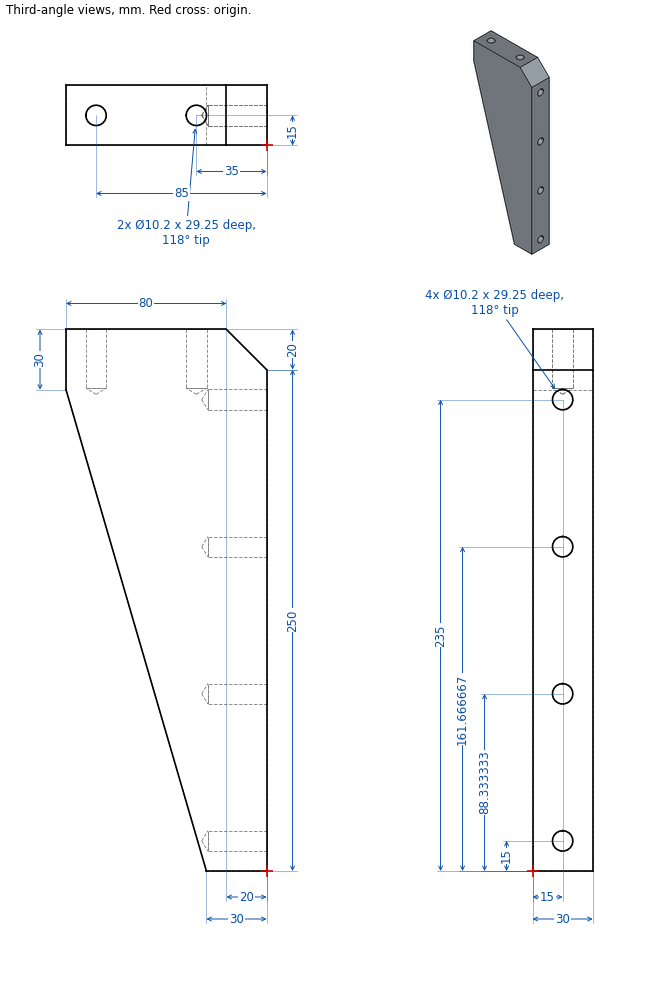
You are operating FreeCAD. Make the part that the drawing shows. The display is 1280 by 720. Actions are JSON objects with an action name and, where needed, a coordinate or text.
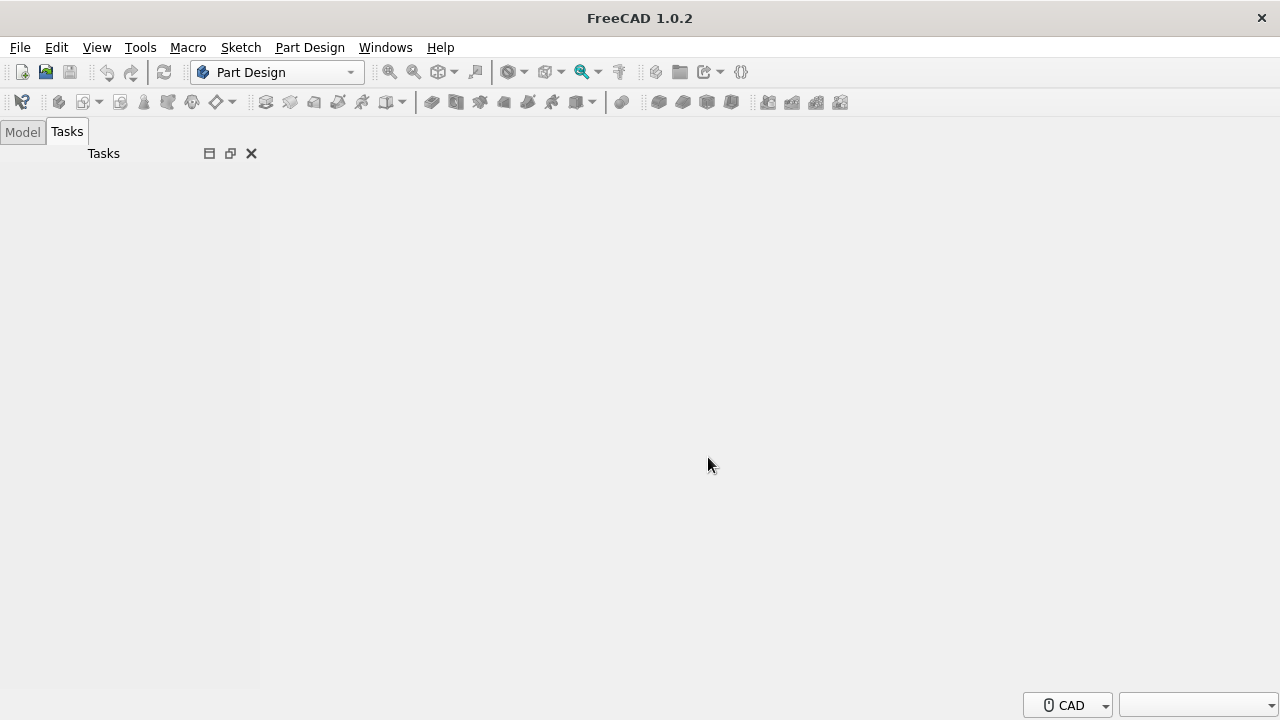
{"action": "key", "text": "ctrl+n"}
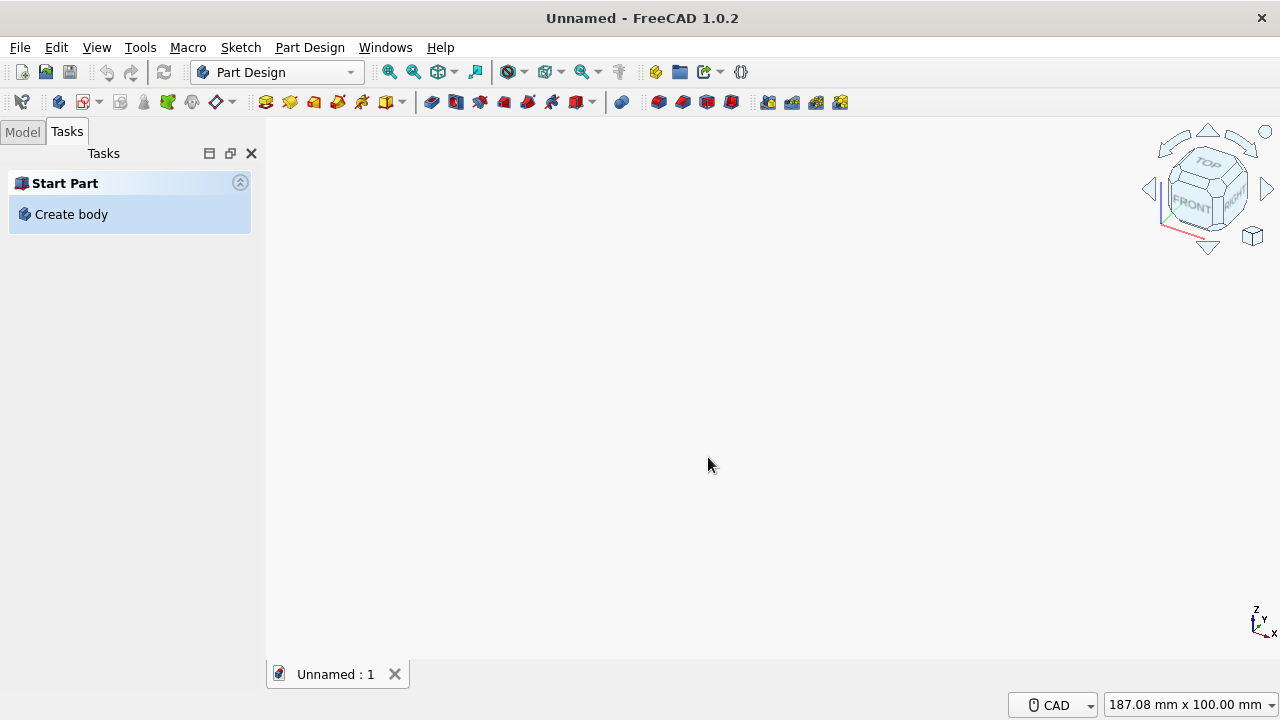
{"action": "left_click", "coordinate": [84, 102]}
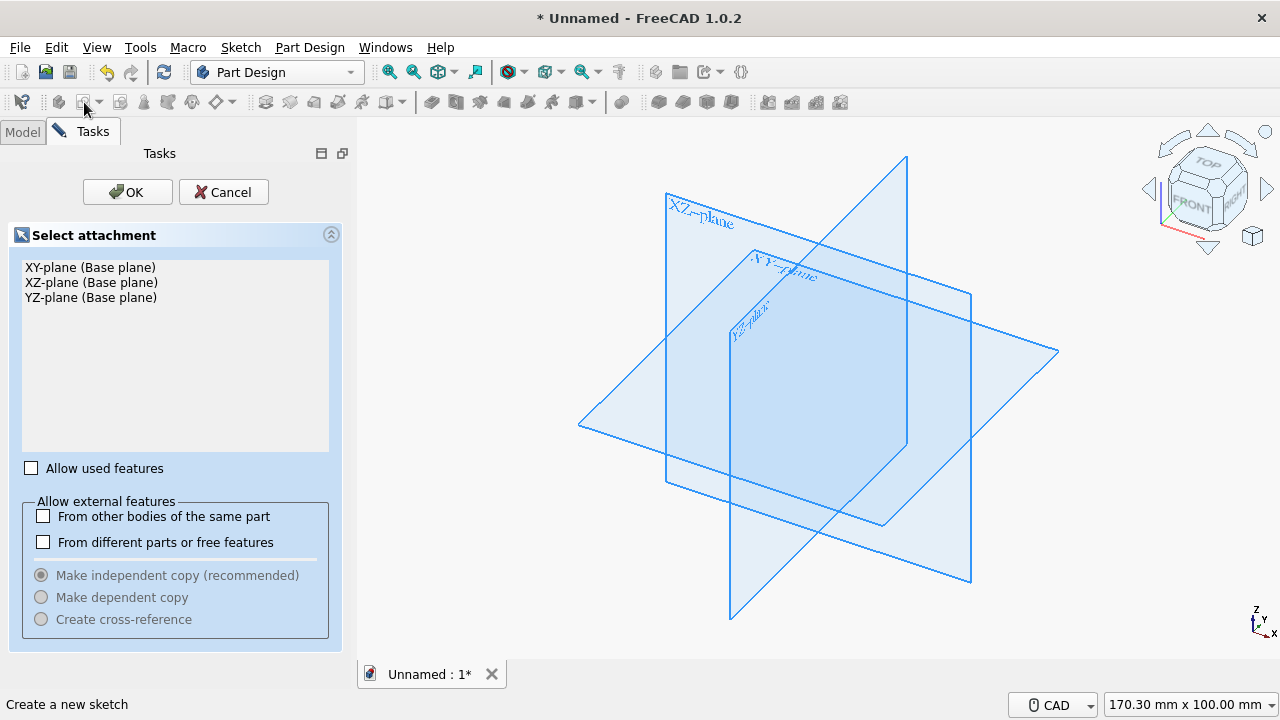
{"action": "left_click", "coordinate": [82, 282]}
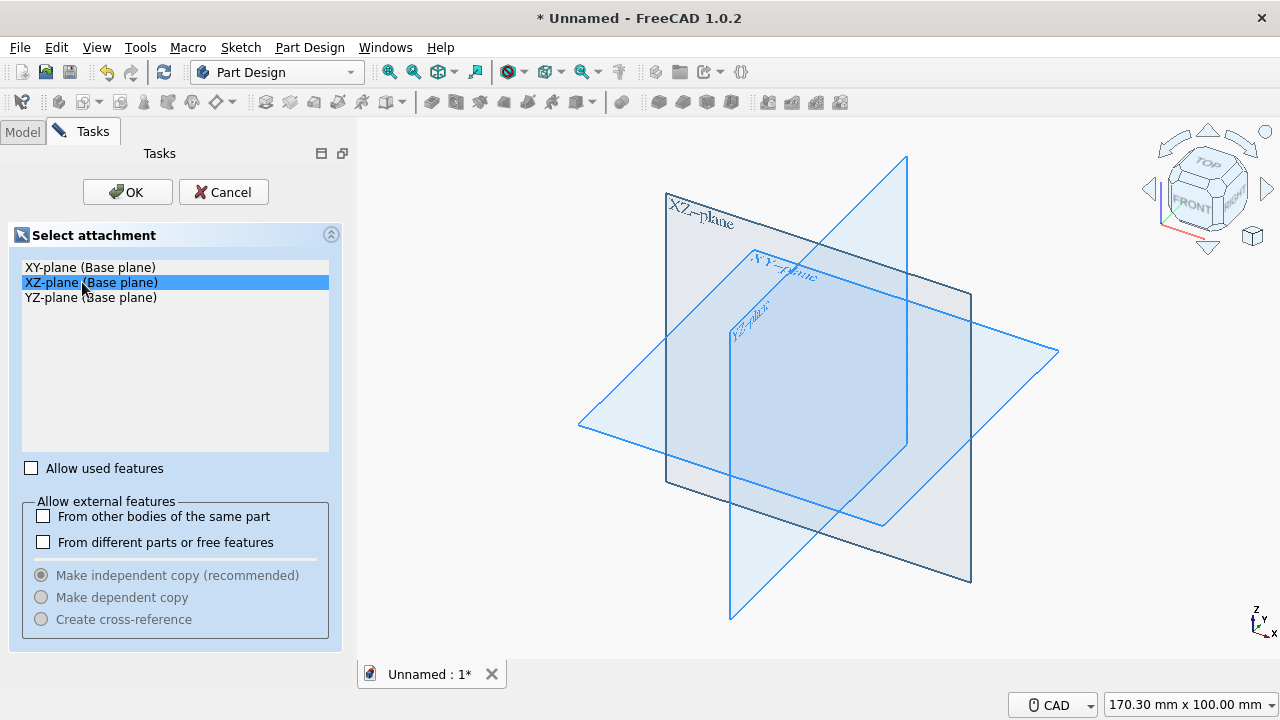
{"action": "left_click", "coordinate": [128, 192]}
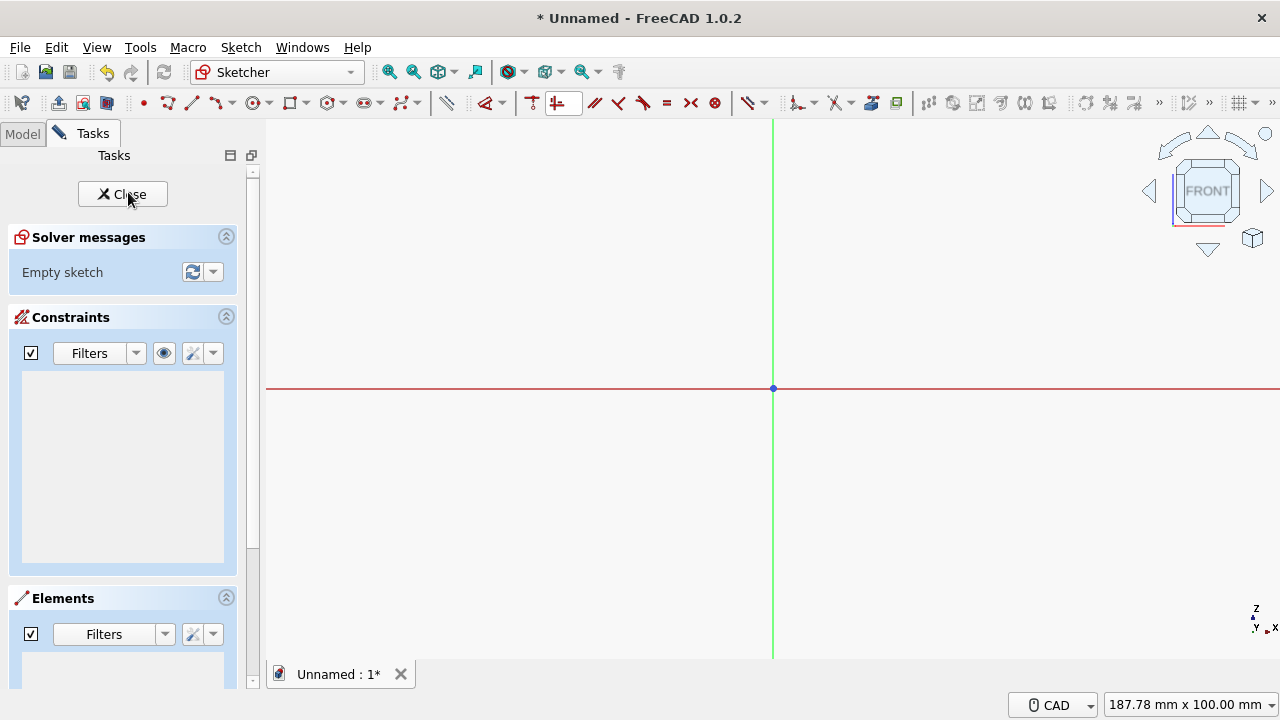
{"action": "scroll", "coordinate": [770, 628], "scroll_direction": "down", "scroll_amount": 7}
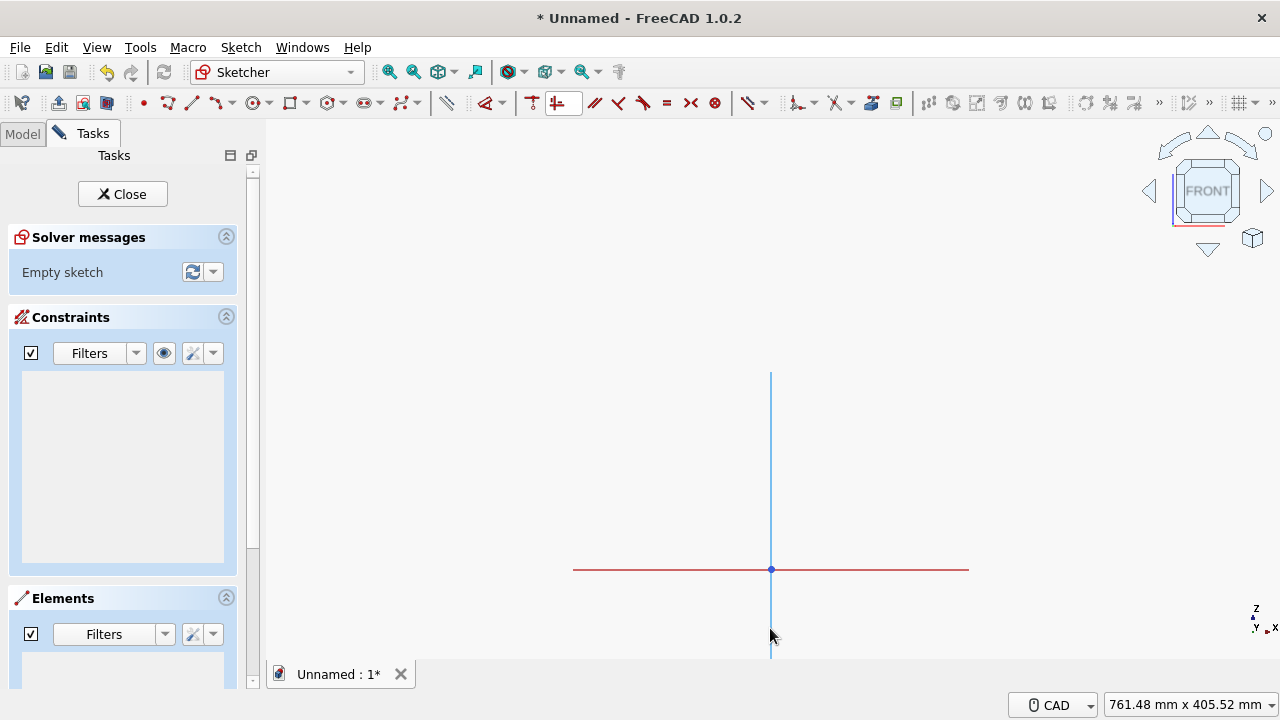
{"action": "key", "text": "g m"}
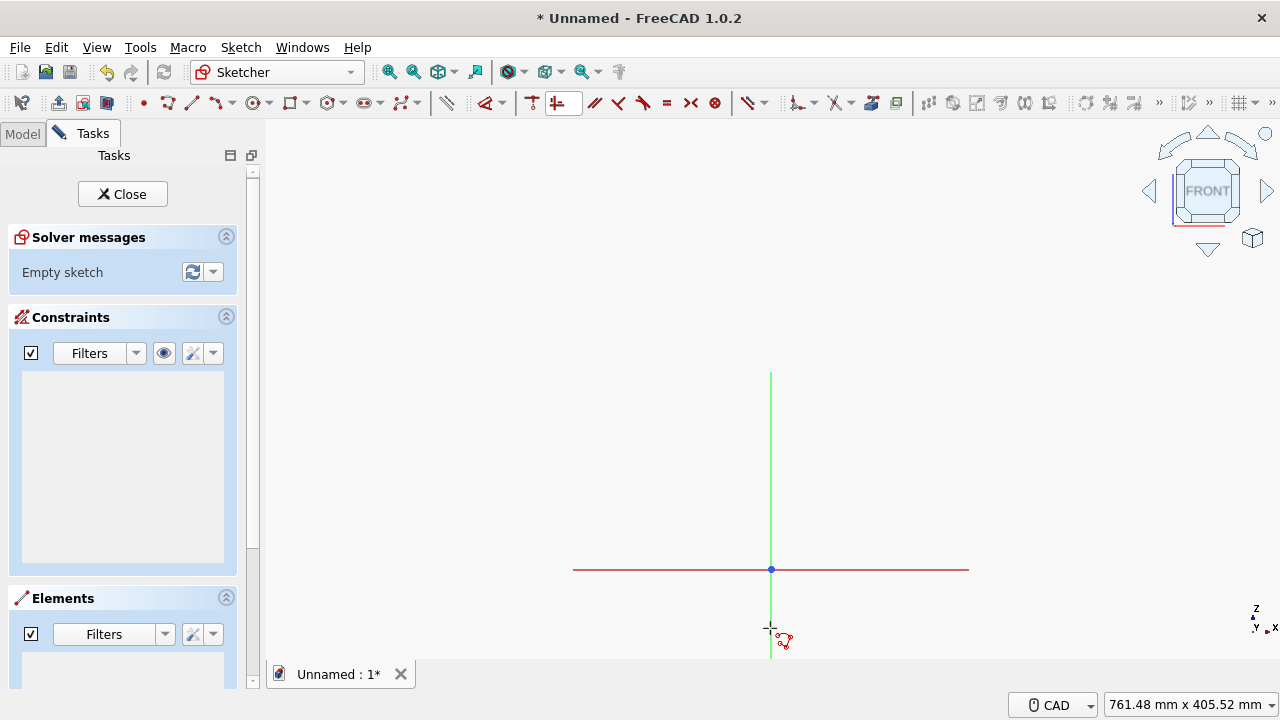
{"action": "left_click", "coordinate": [771, 570]}
{"action": "left_click", "coordinate": [731, 561]}
{"action": "left_click", "coordinate": [638, 250]}
{"action": "left_click", "coordinate": [638, 210]}
{"action": "left_click", "coordinate": [744, 210]}
{"action": "left_click", "coordinate": [762, 237]}
{"action": "left_click", "coordinate": [771, 570]}
{"action": "key", "text": "Escape"}
{"action": "key", "text": "Escape"}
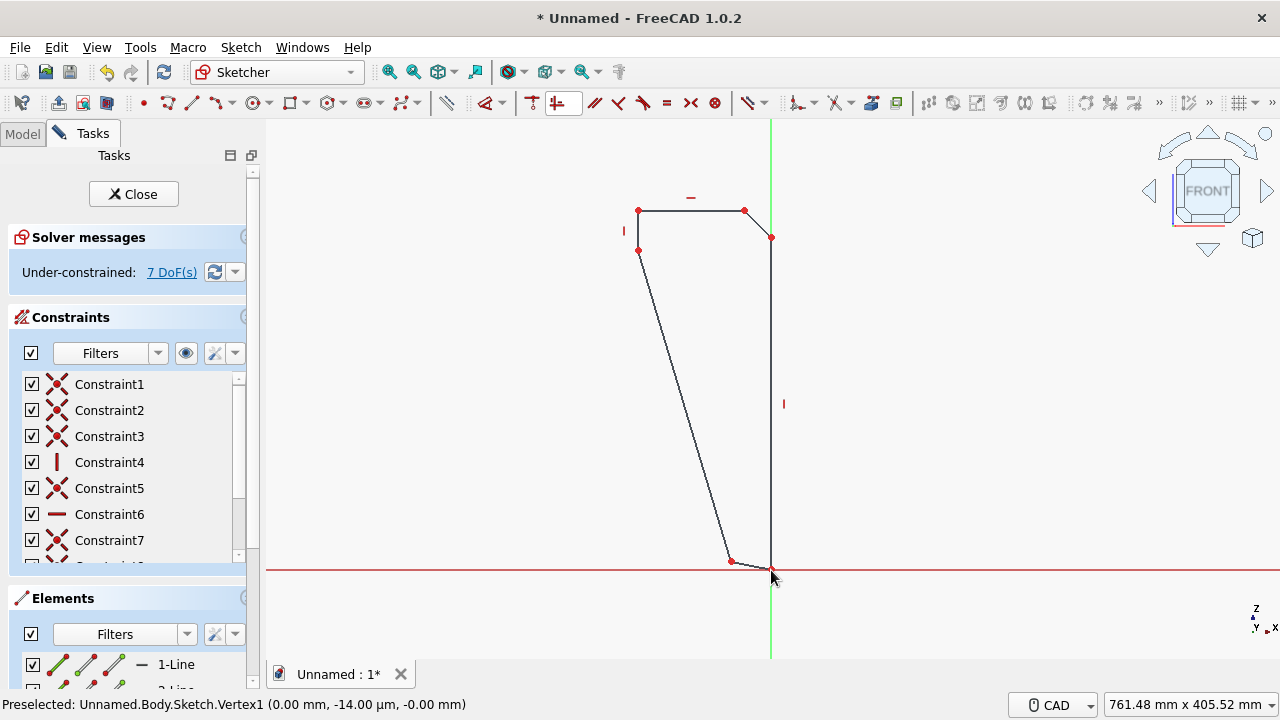
{"action": "left_click", "coordinate": [759, 567]}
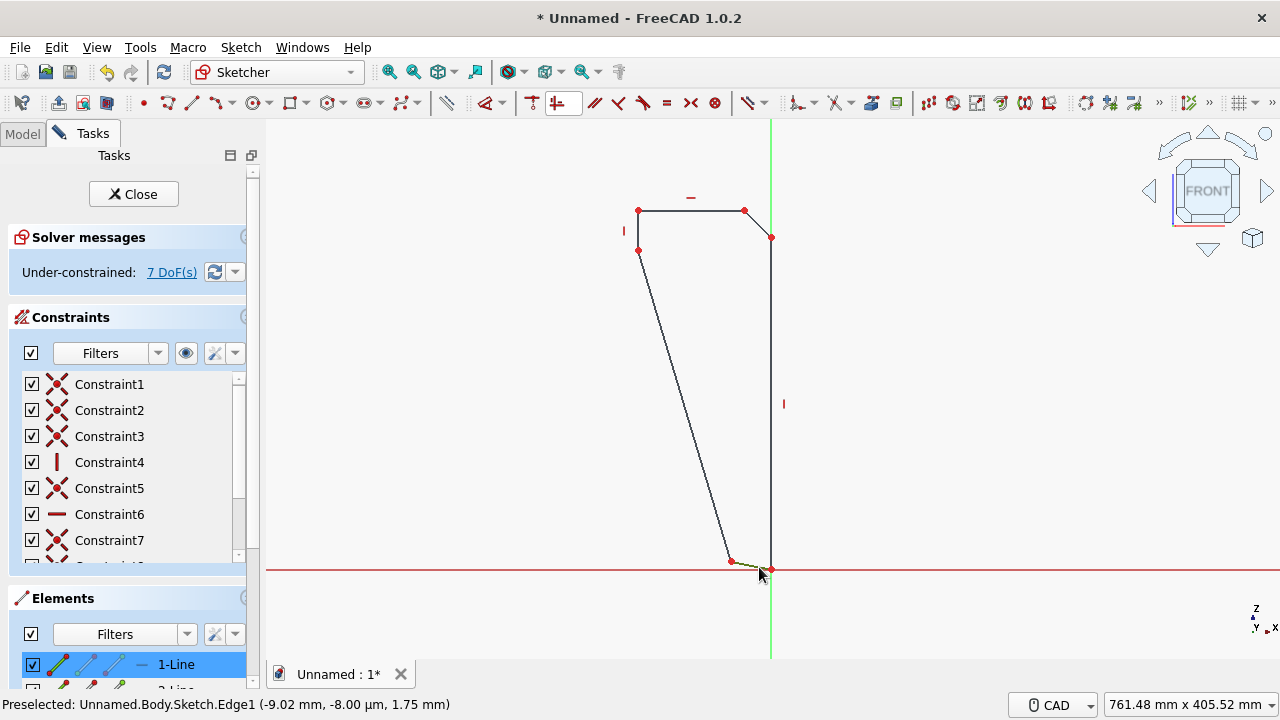
{"action": "key", "text": "h"}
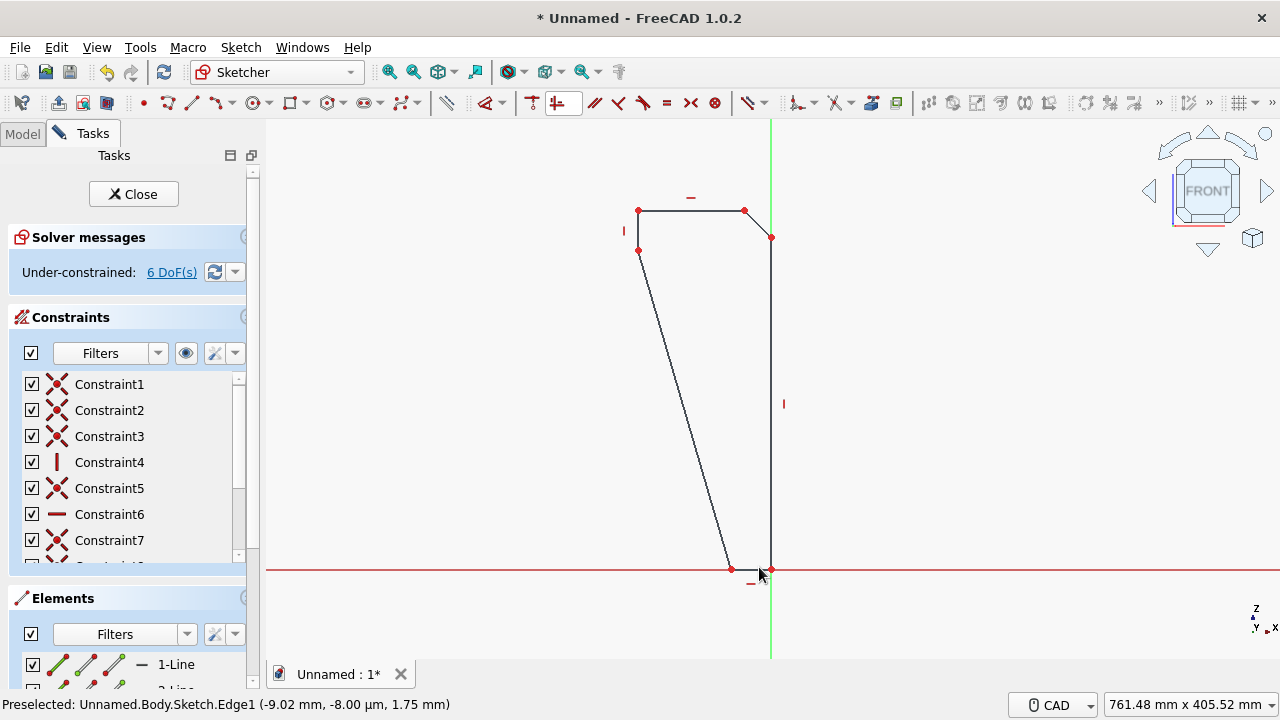
{"action": "left_click", "coordinate": [486, 104]}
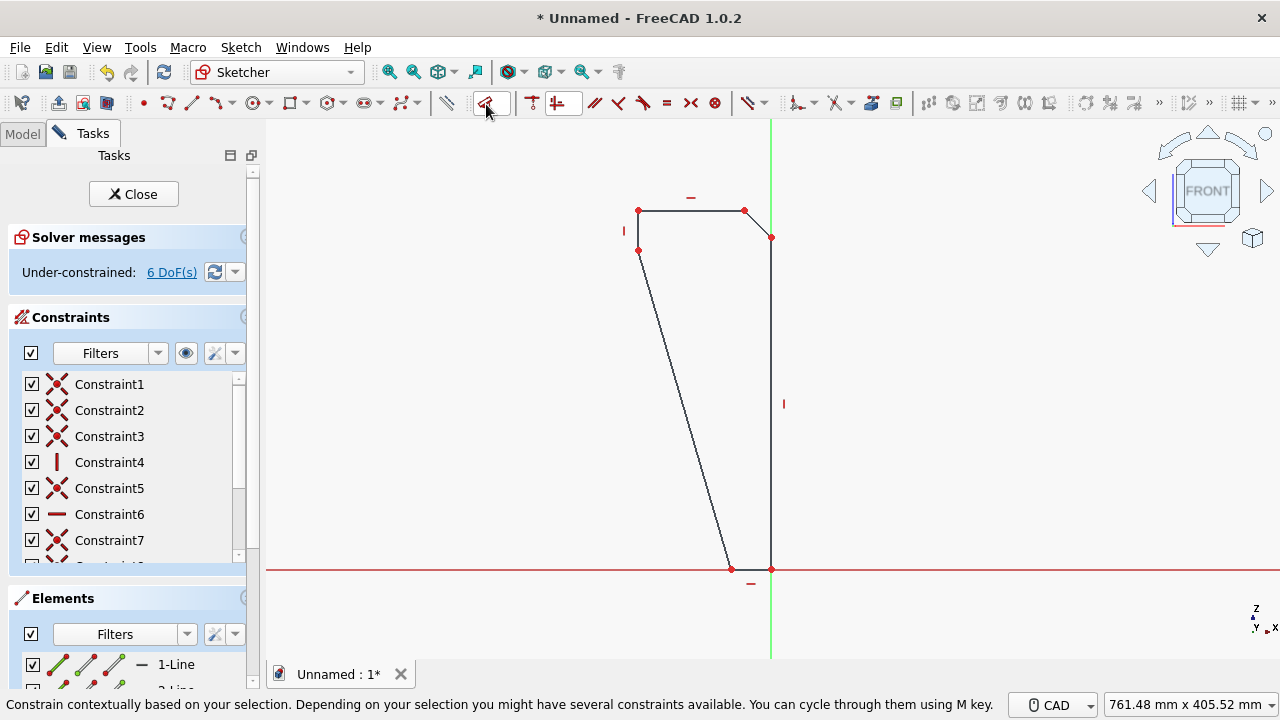
{"action": "left_click", "coordinate": [759, 570]}
{"action": "left_click", "coordinate": [751, 604]}